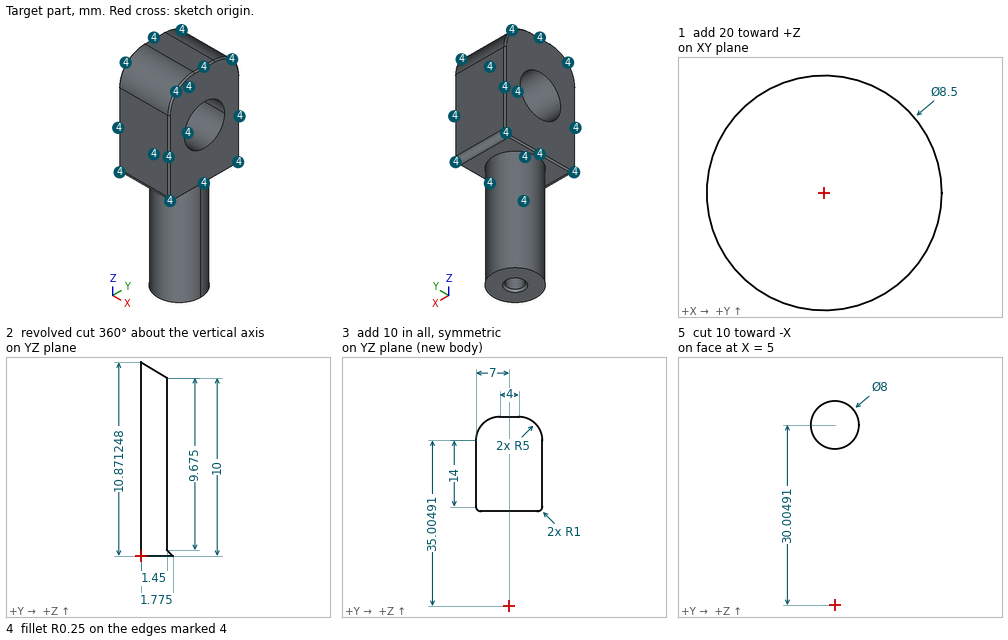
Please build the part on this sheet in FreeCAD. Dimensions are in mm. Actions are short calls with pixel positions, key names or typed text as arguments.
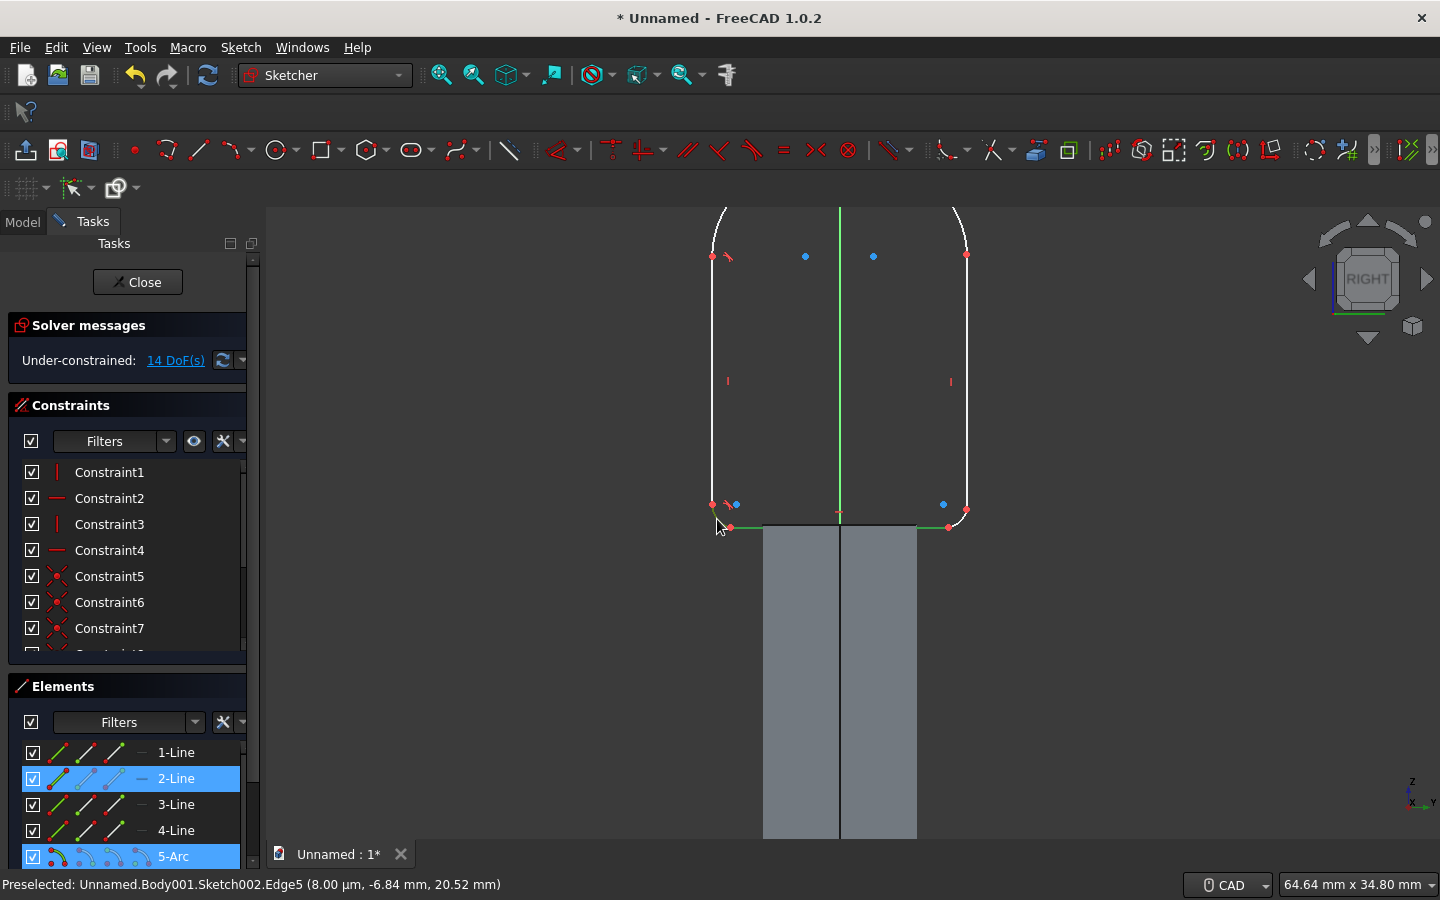
key(t)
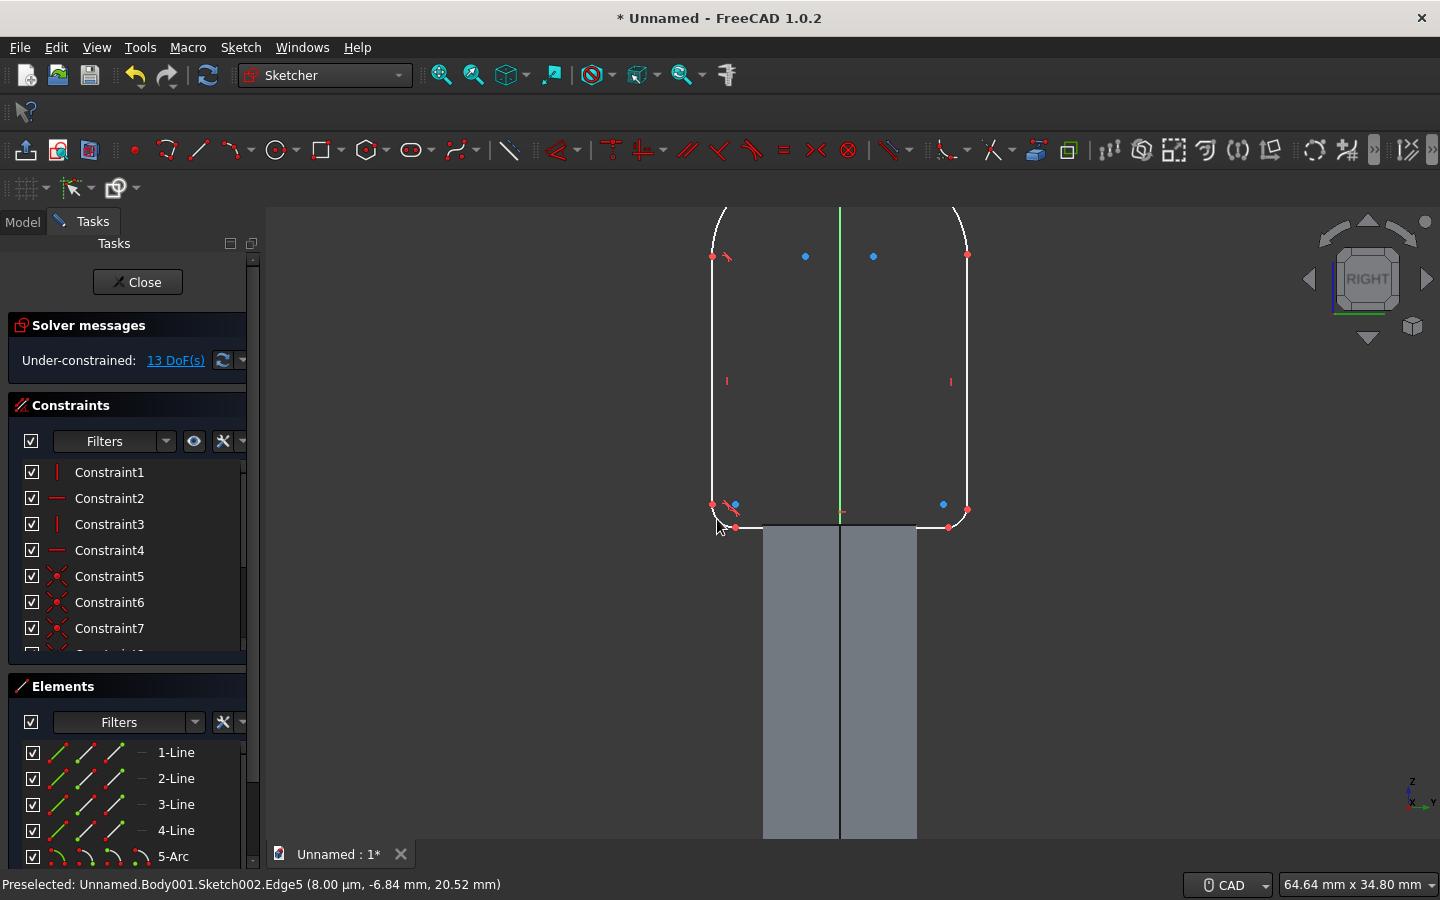
click(799, 528)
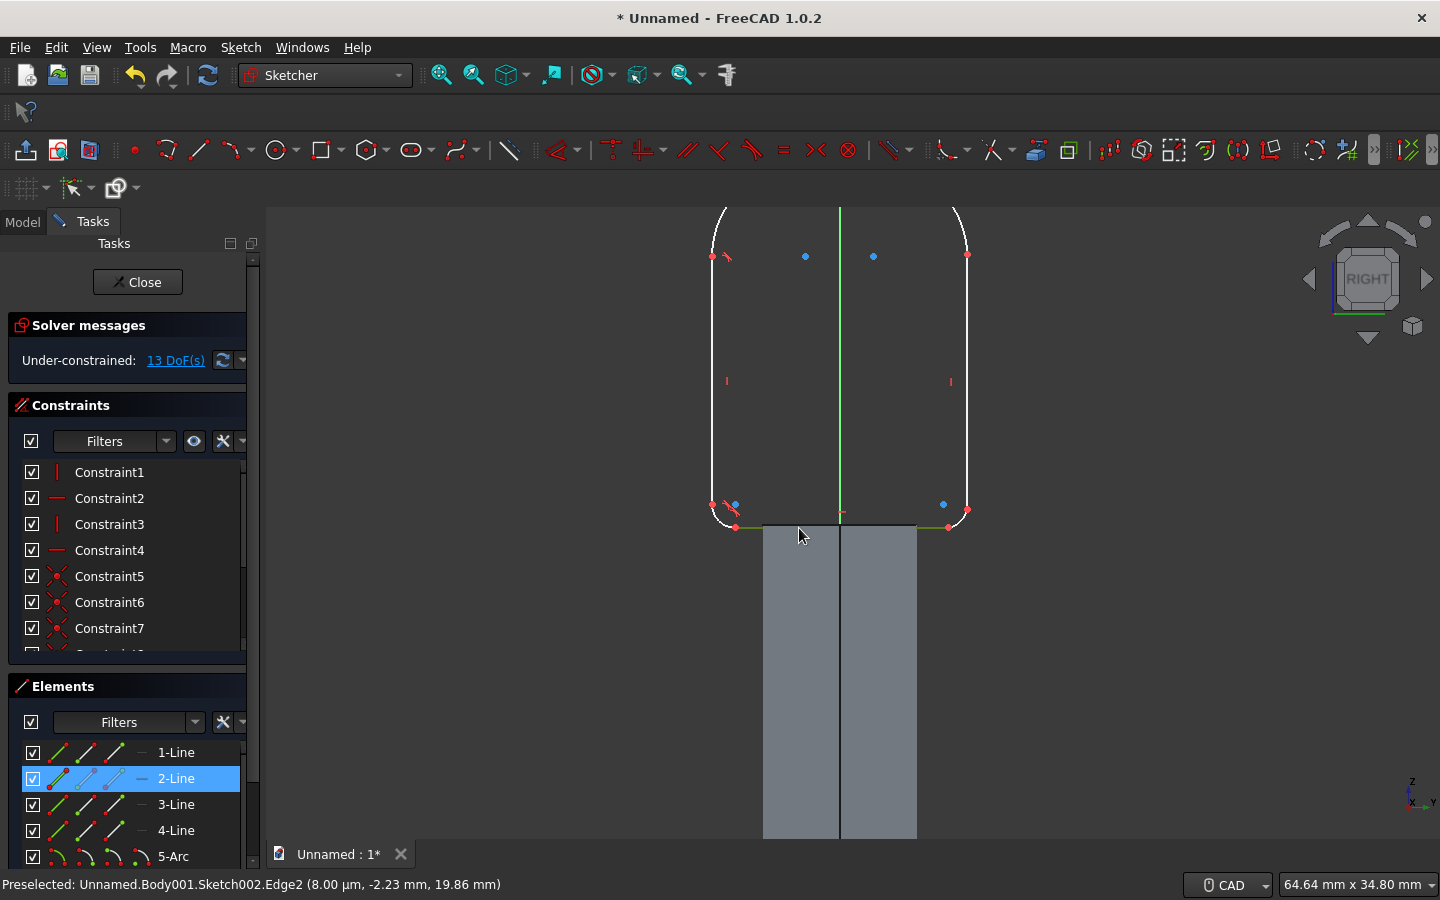
click(961, 521)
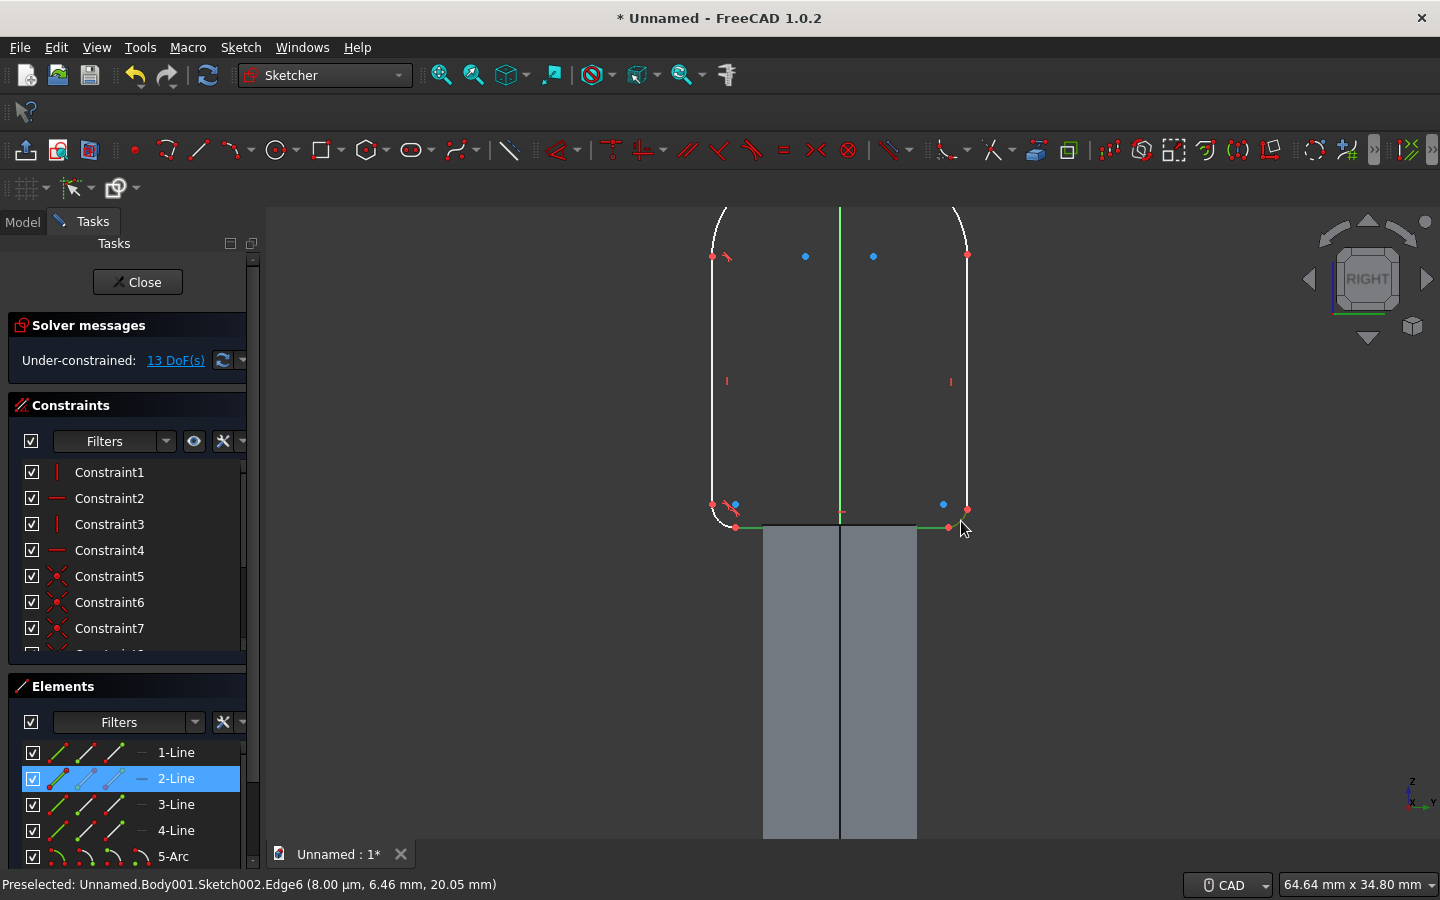
click(752, 150)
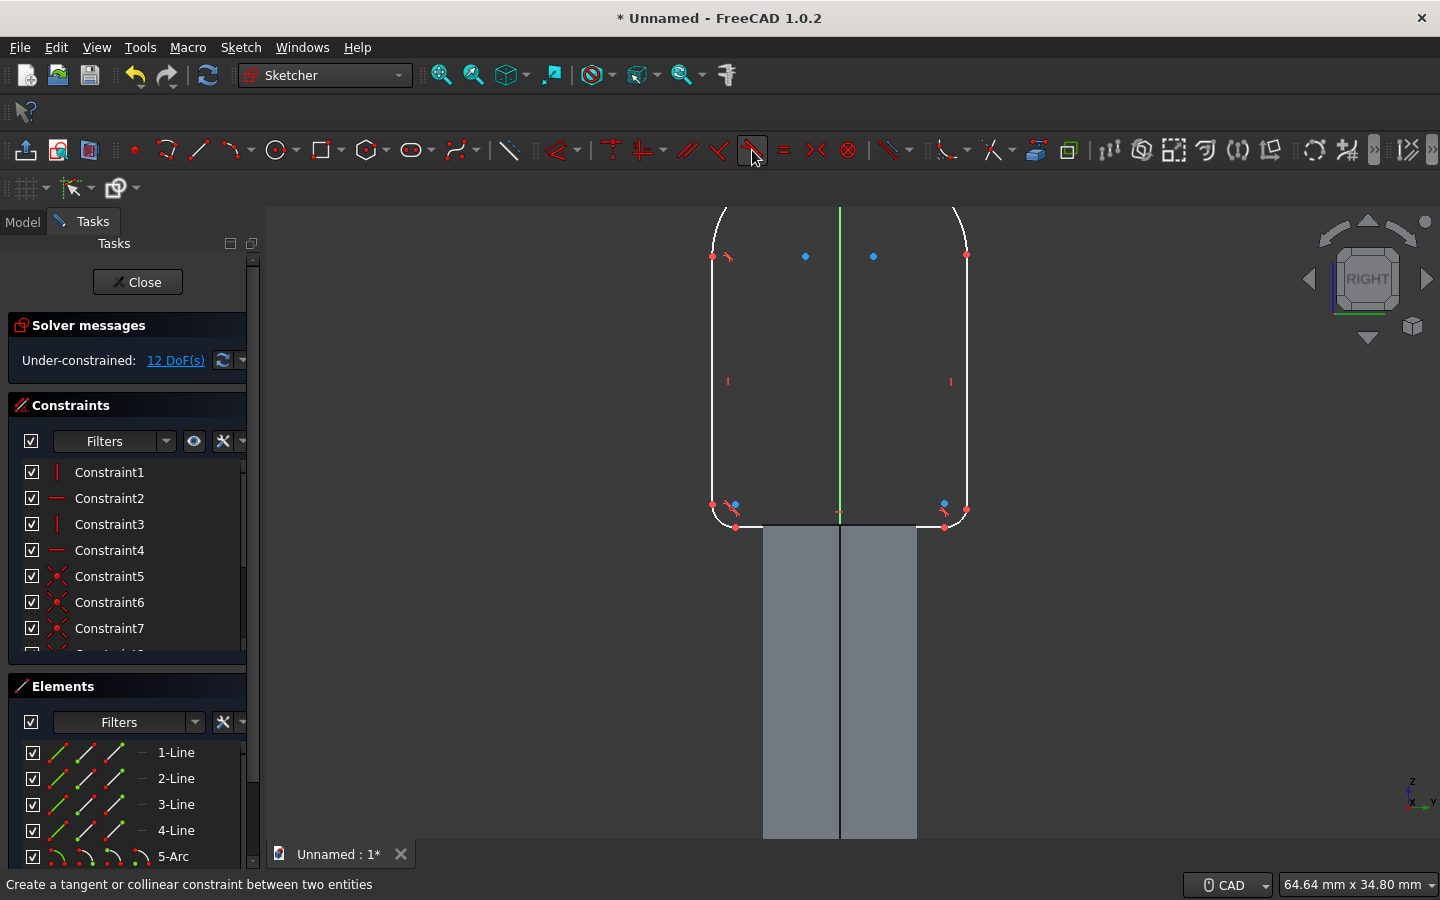
click(967, 433)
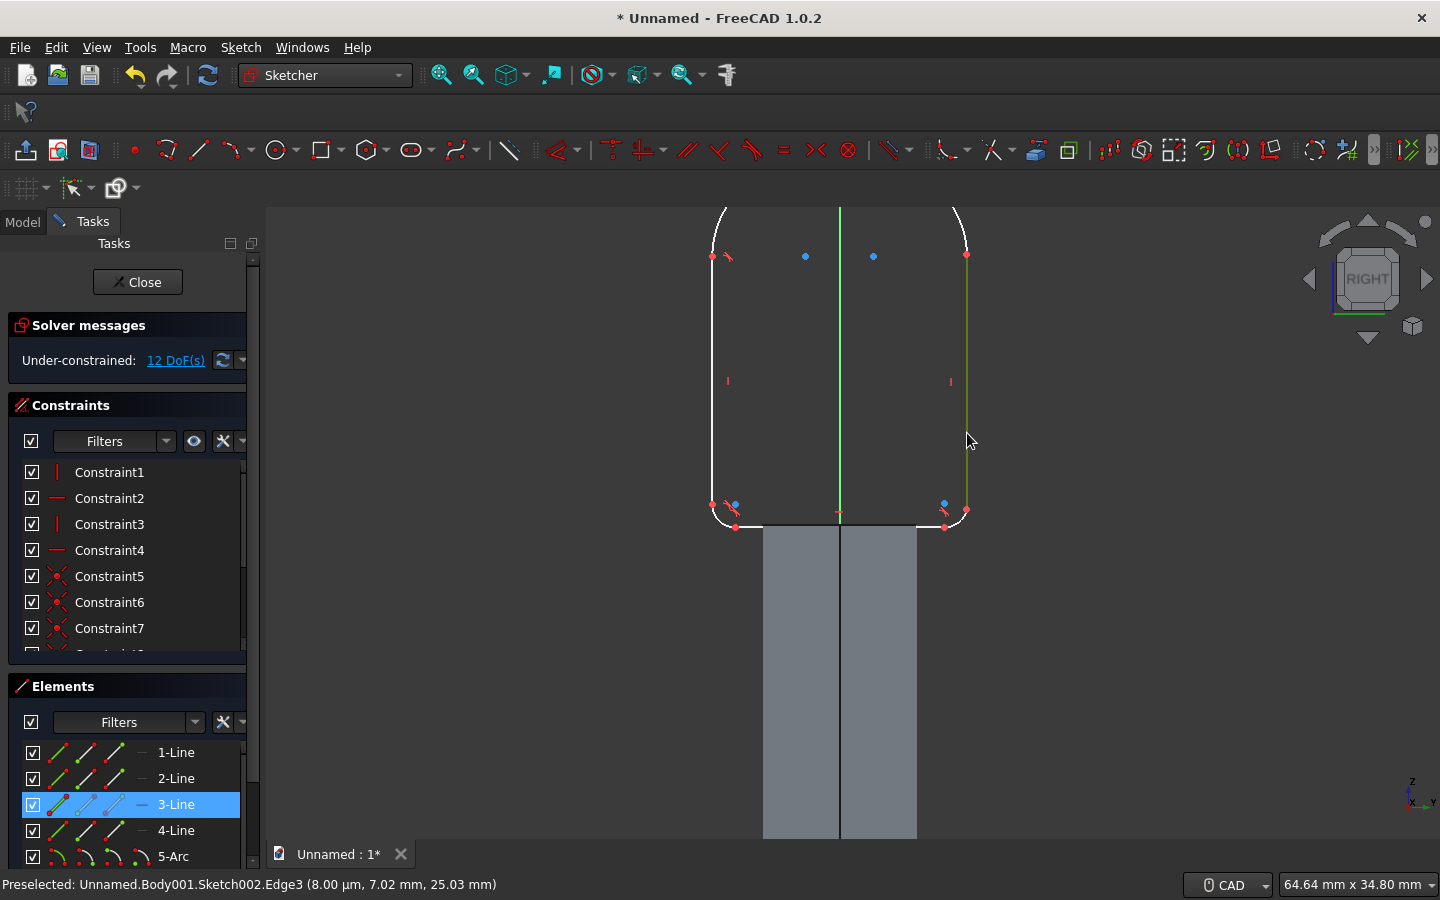
scroll(953, 526, up, 2)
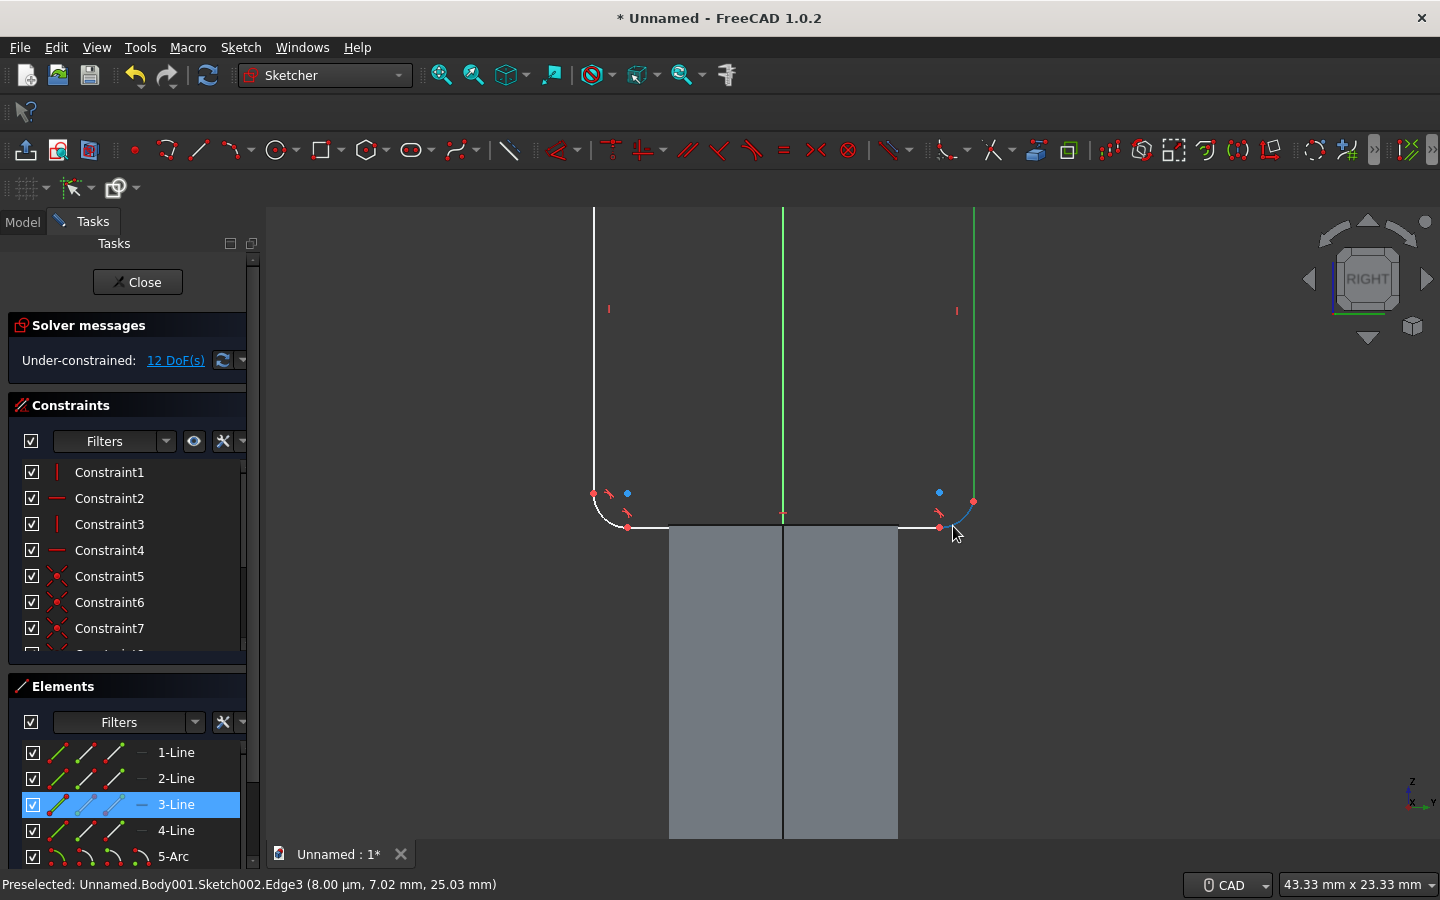
click(953, 525)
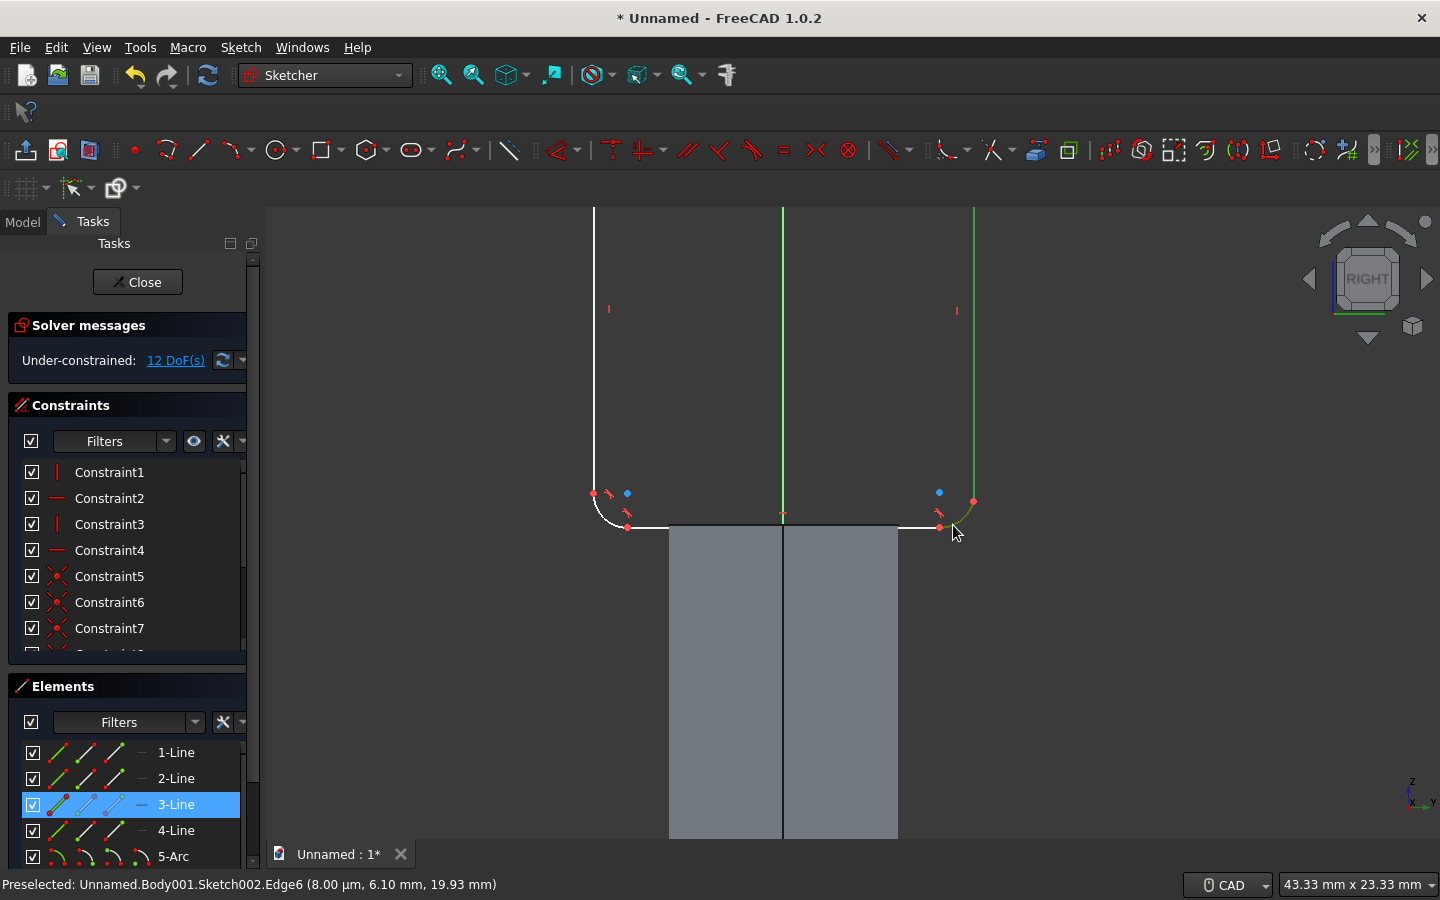
click(752, 150)